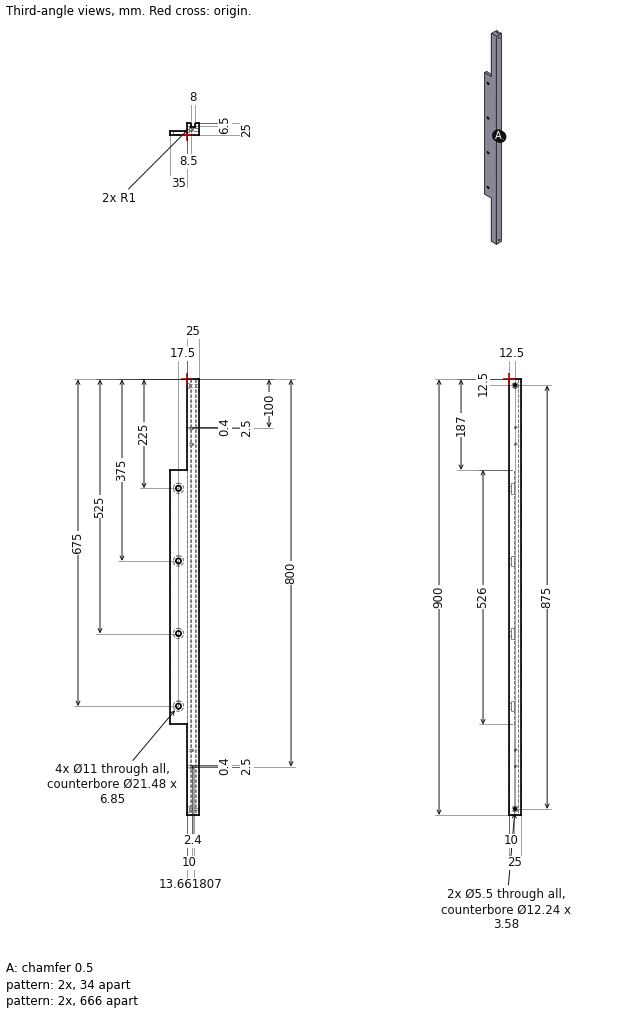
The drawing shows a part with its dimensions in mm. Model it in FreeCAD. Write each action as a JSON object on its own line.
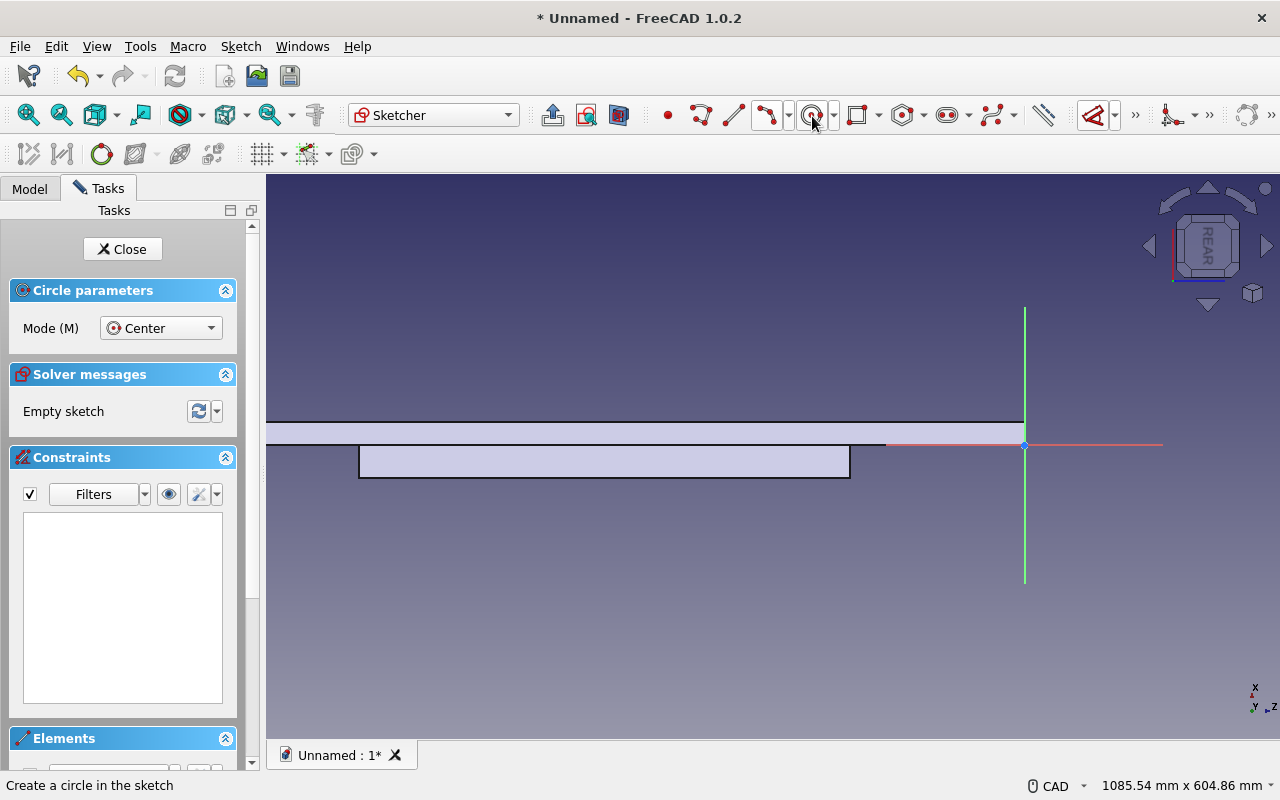
{"action": "scroll", "coordinate": [394, 462], "scroll_direction": "up", "scroll_amount": 8}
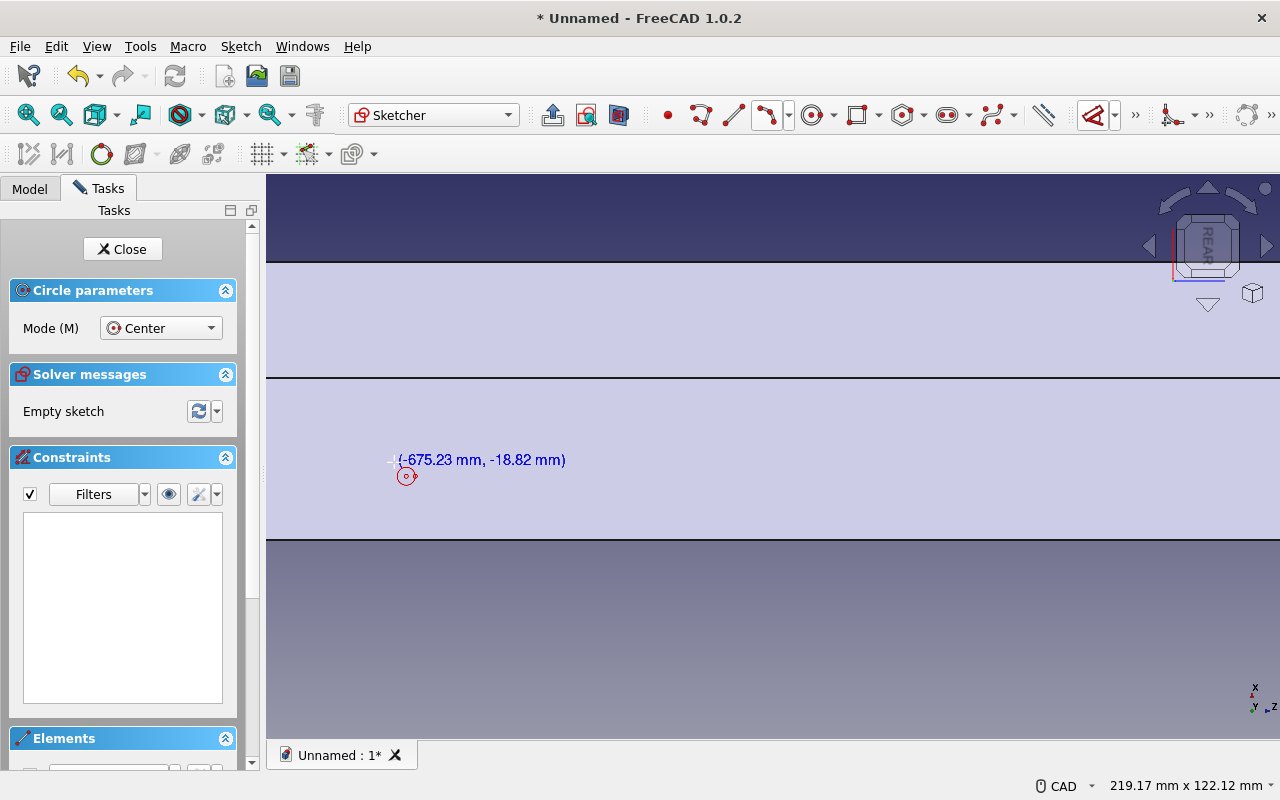
{"action": "scroll", "coordinate": [391, 463], "scroll_direction": "down", "scroll_amount": 8}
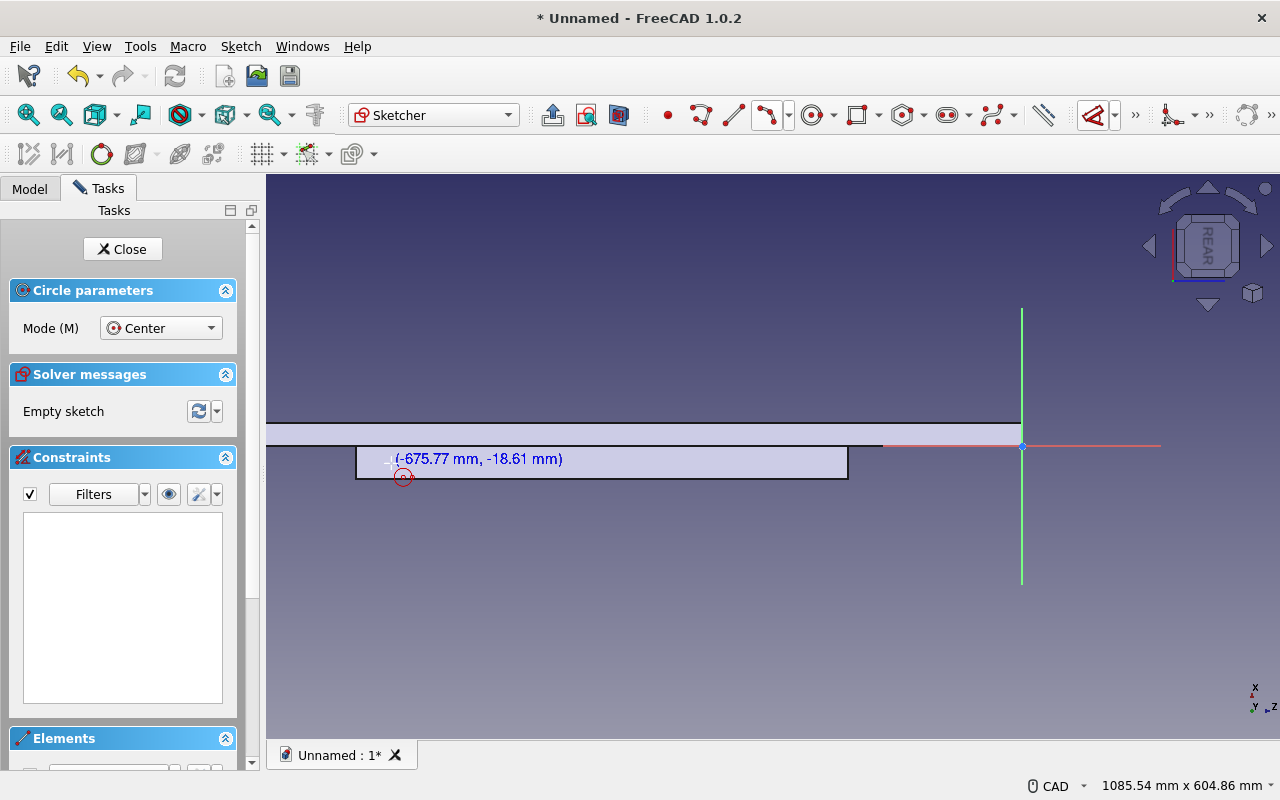
{"action": "left_click", "coordinate": [392, 463]}
{"action": "mouse_move", "coordinate": [395, 466]}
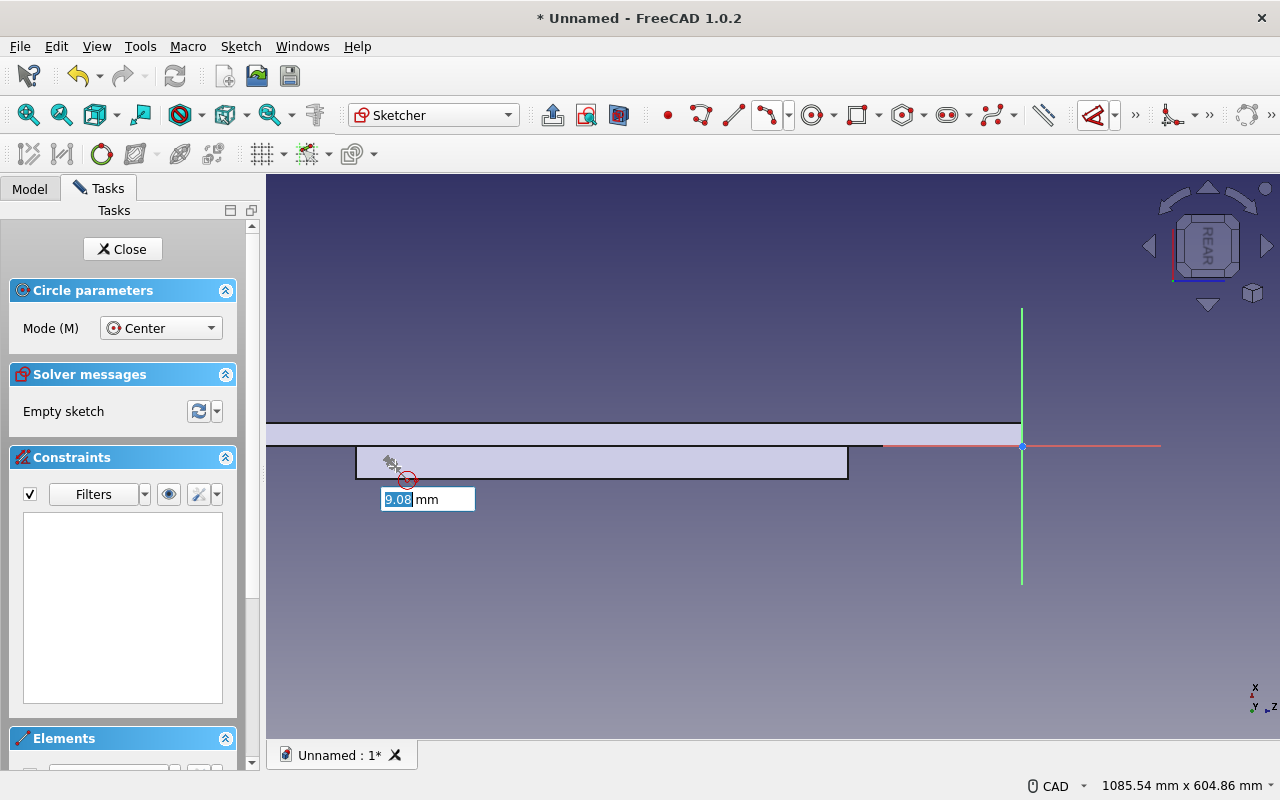
{"action": "type", "text": "11"}
{"action": "key", "text": "Return"}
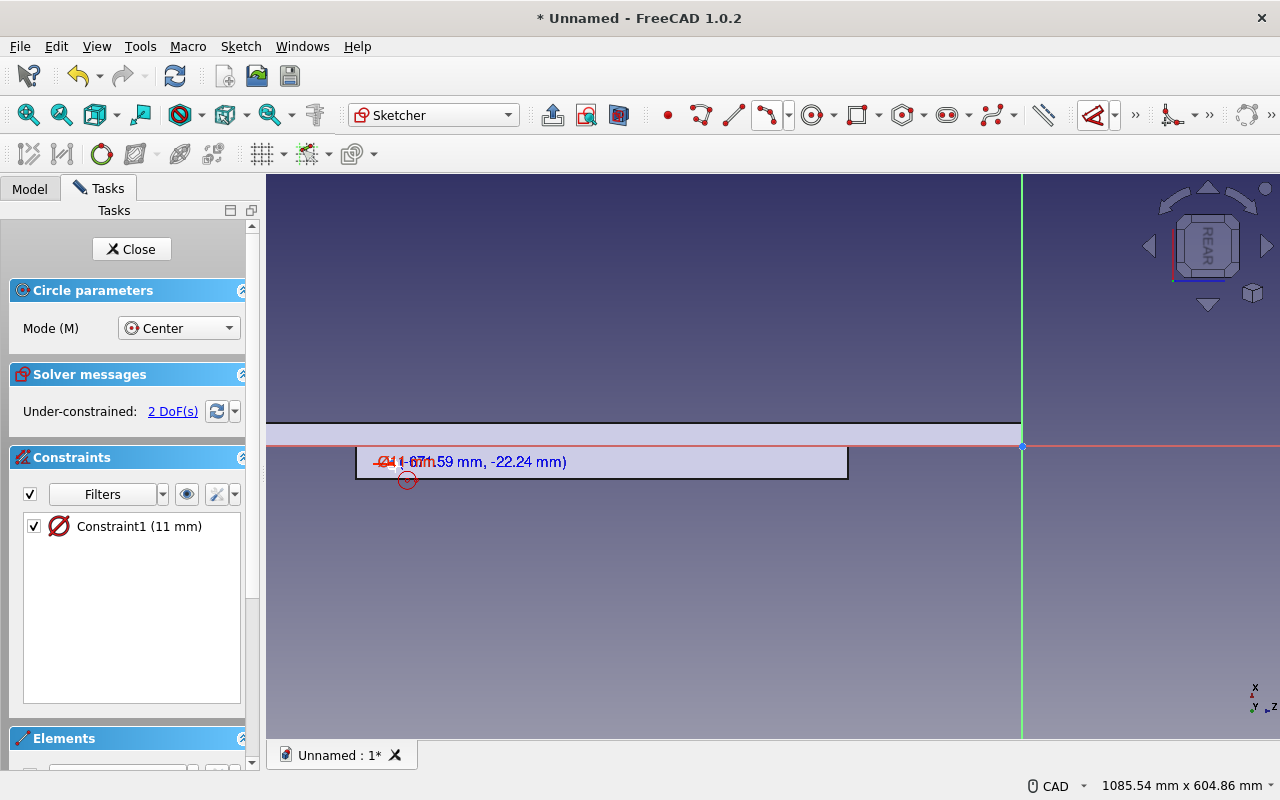
{"action": "scroll", "coordinate": [532, 463], "scroll_direction": "up", "scroll_amount": 8}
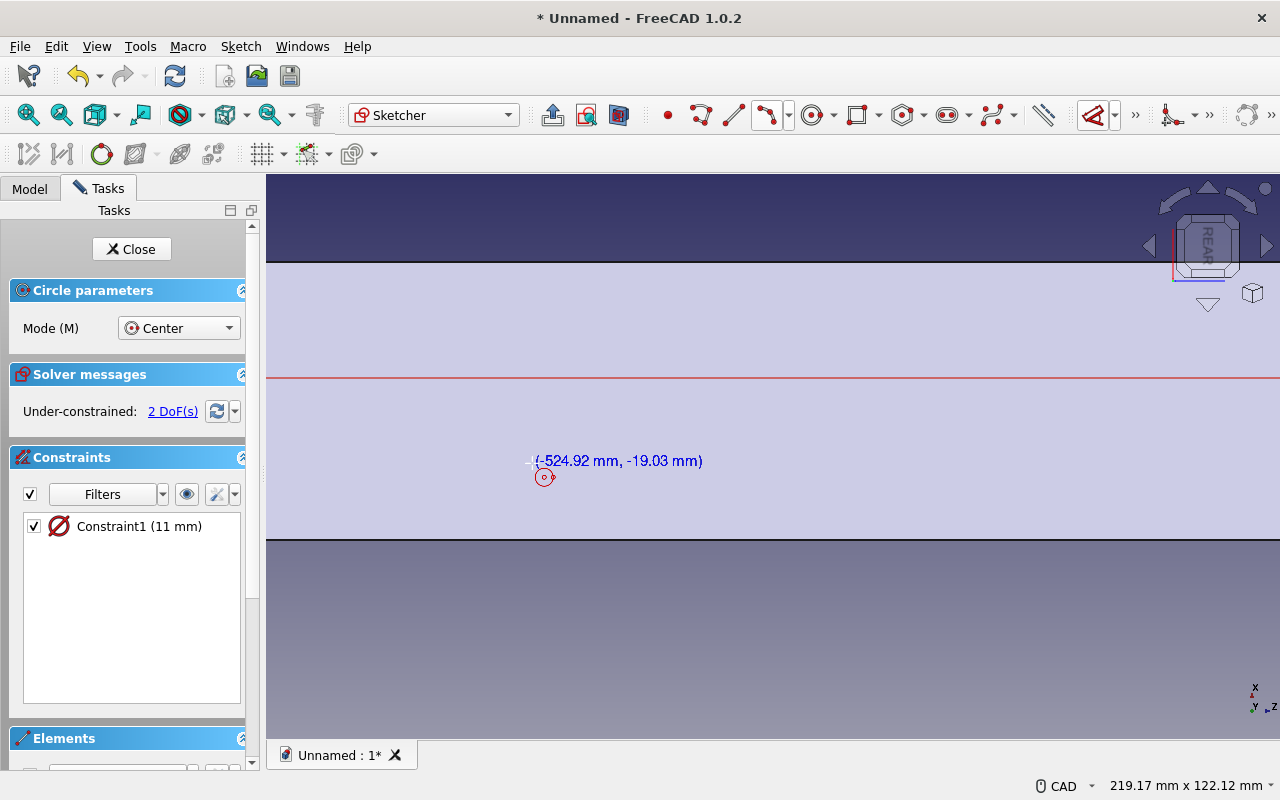
{"action": "scroll", "coordinate": [532, 463], "scroll_direction": "down", "scroll_amount": 8}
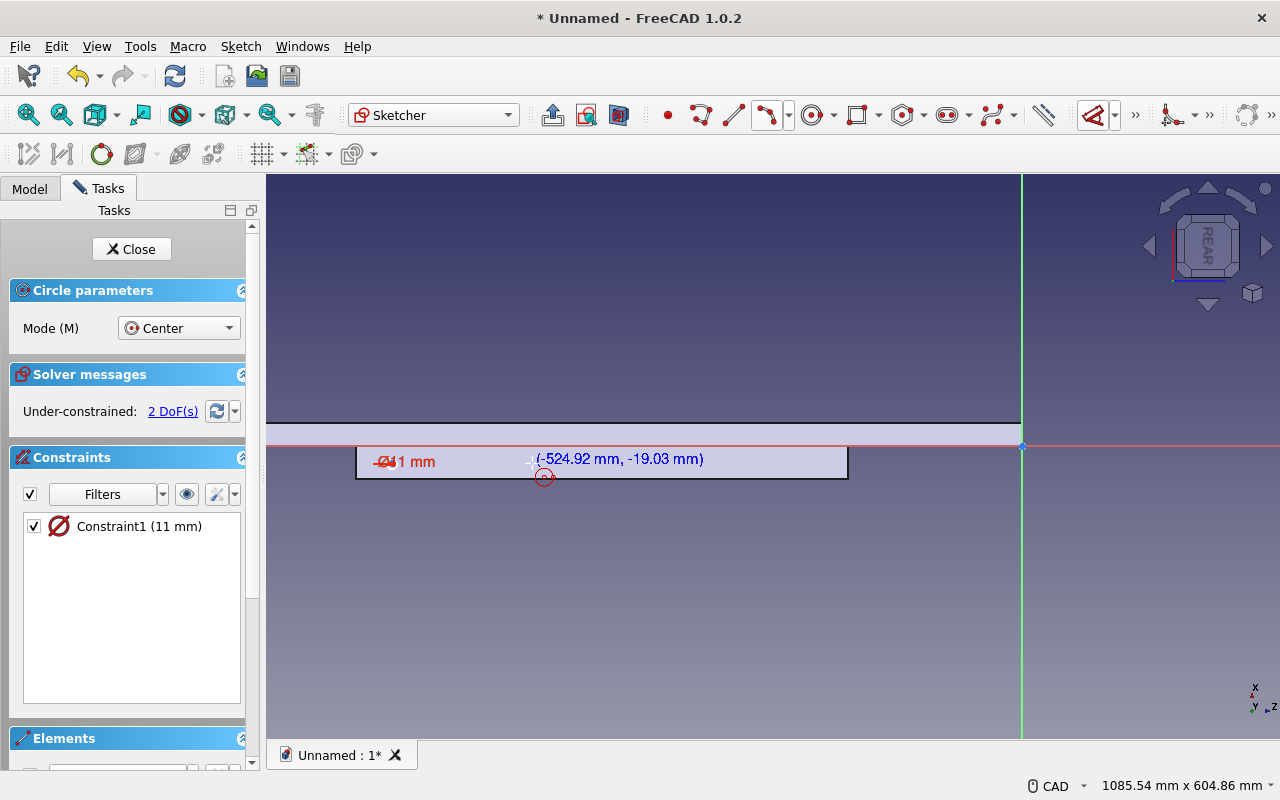
{"action": "left_click", "coordinate": [532, 463]}
{"action": "mouse_move", "coordinate": [536, 466]}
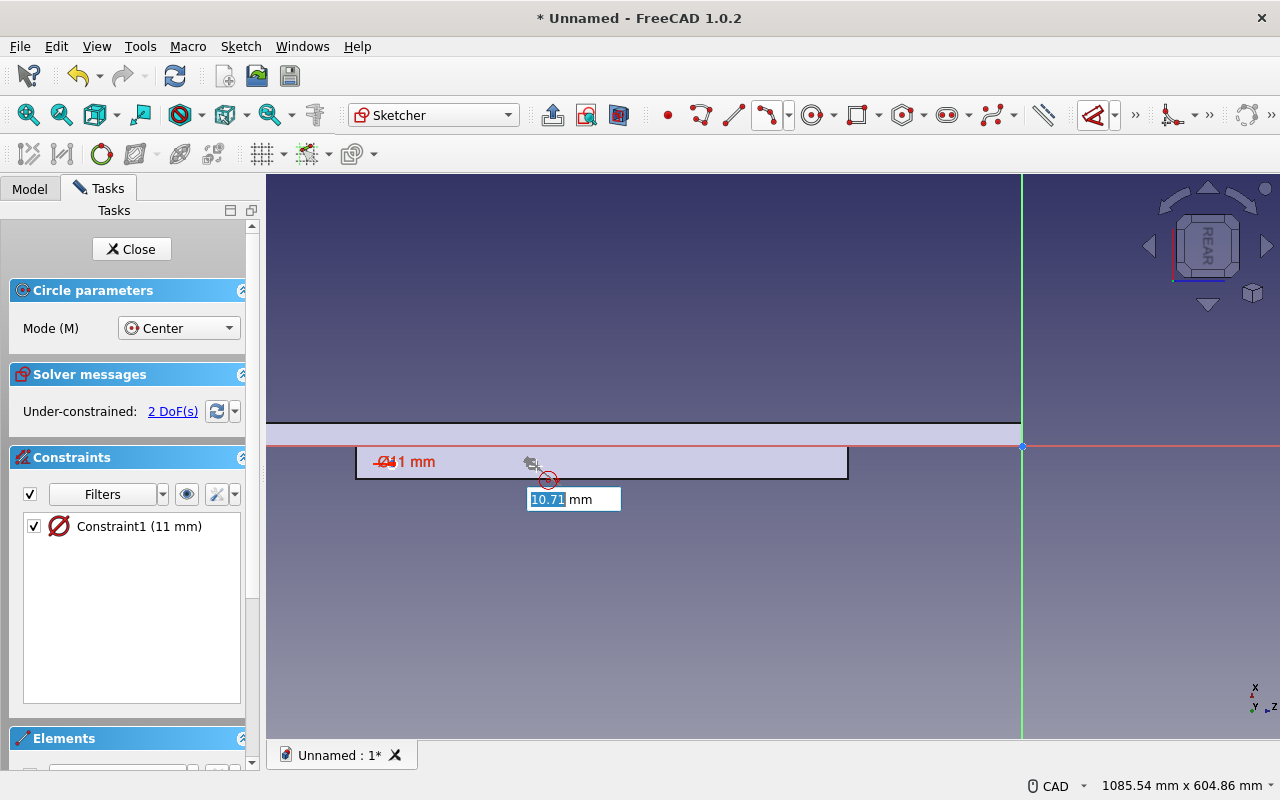
{"action": "type", "text": "11"}
{"action": "key", "text": "Return"}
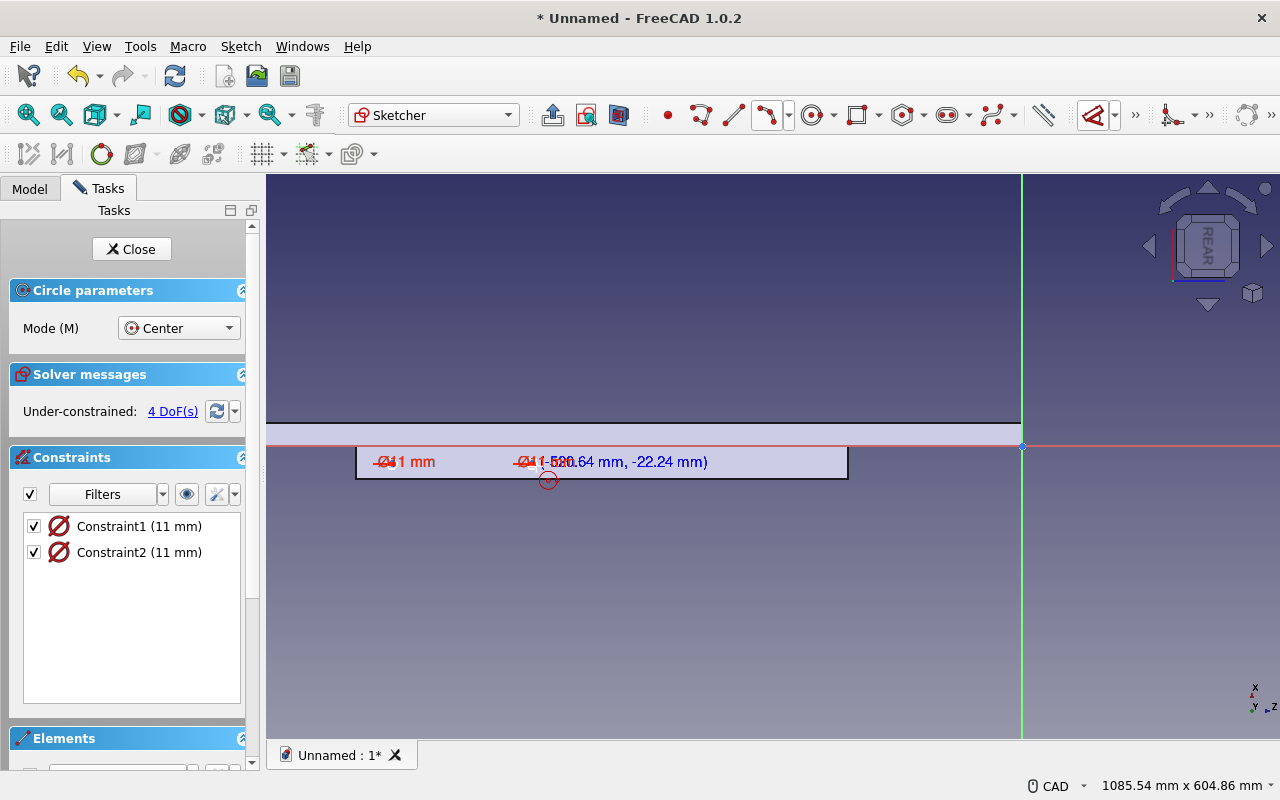
{"action": "scroll", "coordinate": [672, 463], "scroll_direction": "up", "scroll_amount": 8}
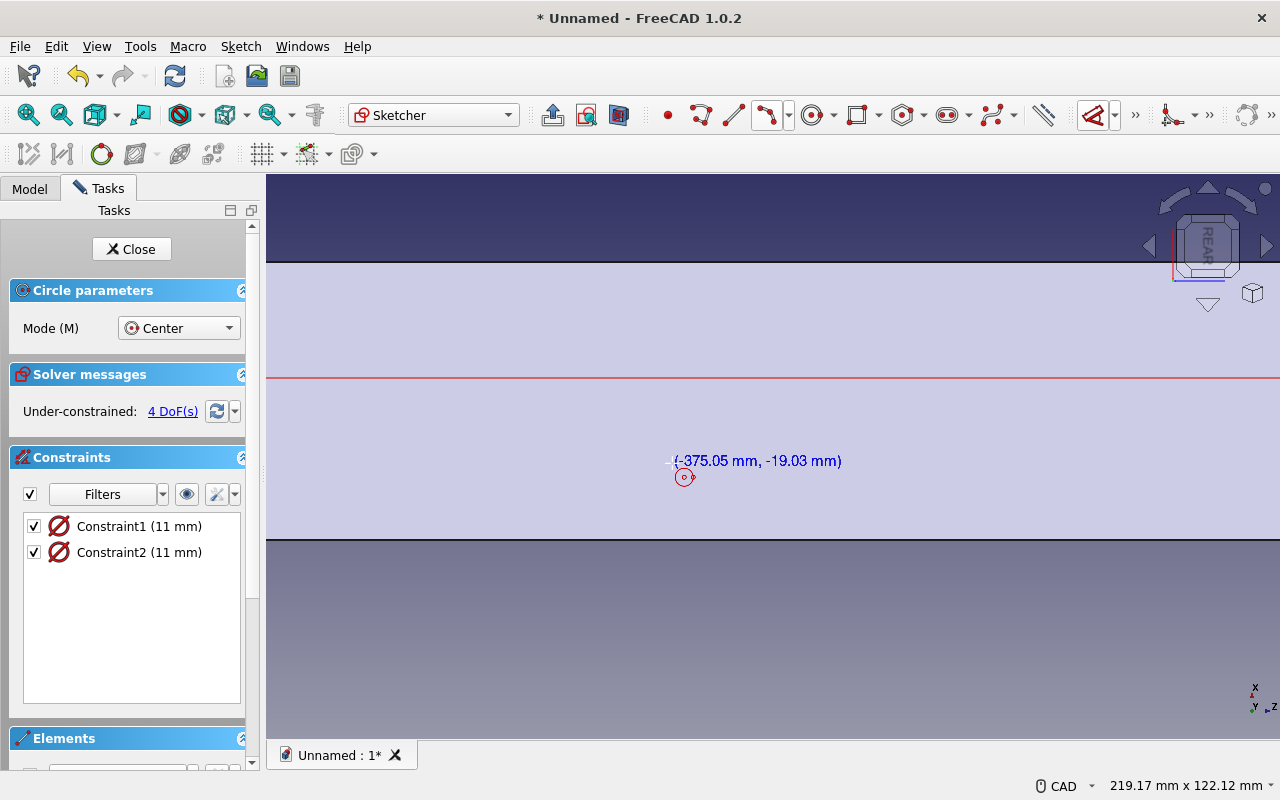
{"action": "scroll", "coordinate": [672, 463], "scroll_direction": "down", "scroll_amount": 8}